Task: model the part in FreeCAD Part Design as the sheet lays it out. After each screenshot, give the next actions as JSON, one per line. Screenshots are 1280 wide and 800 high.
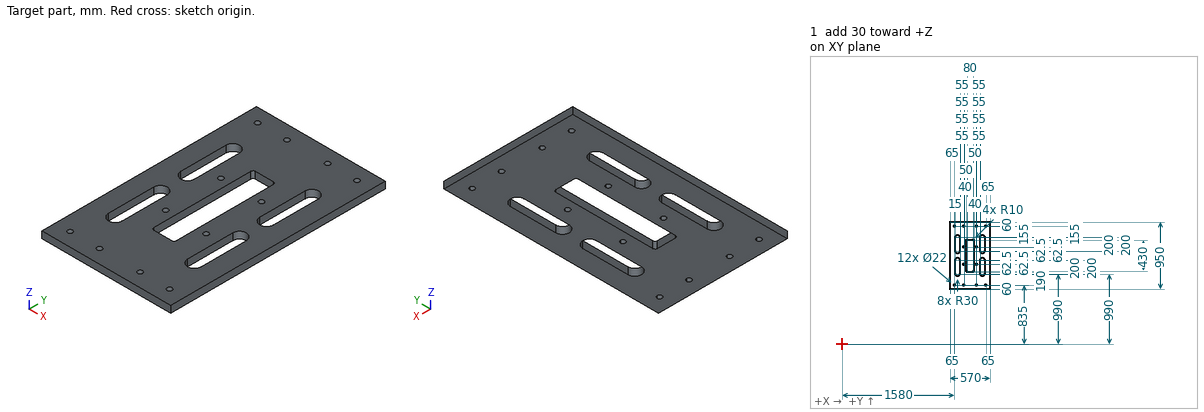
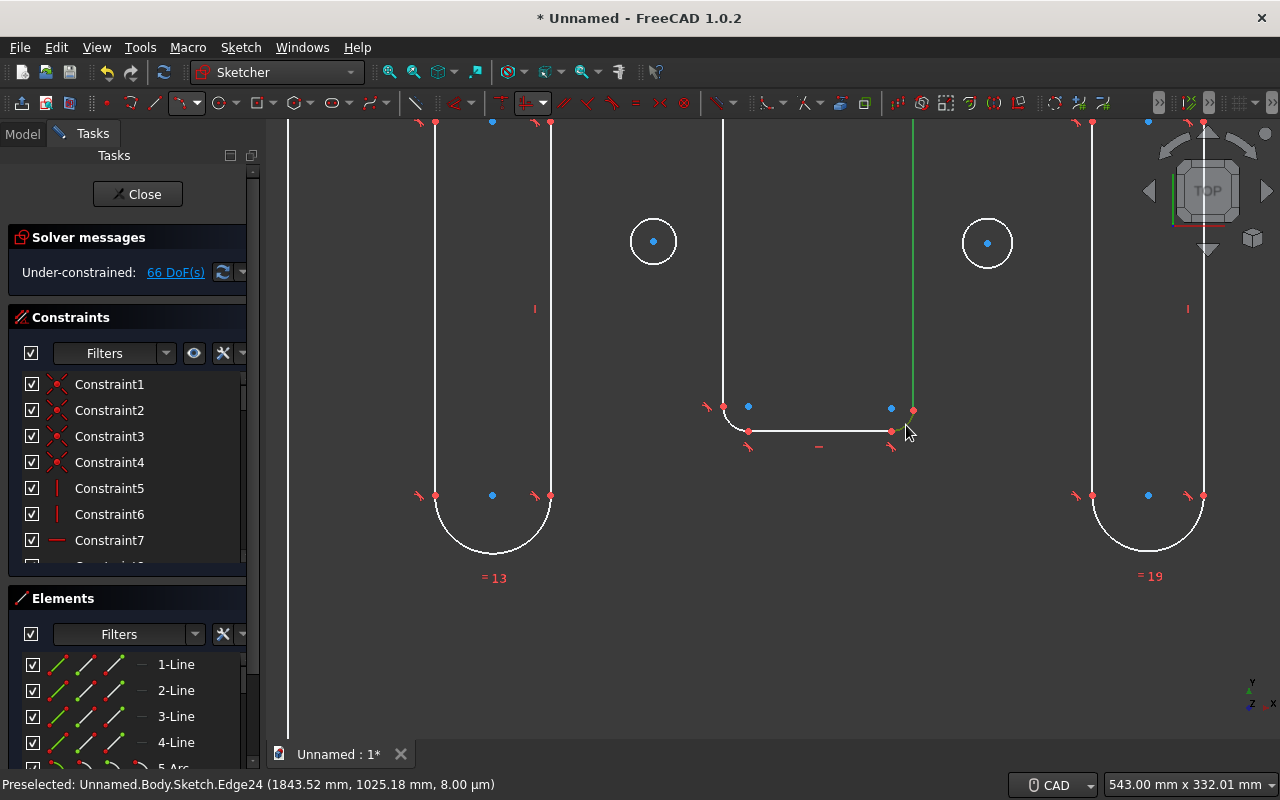
{"action": "left_click", "coordinate": [612, 104]}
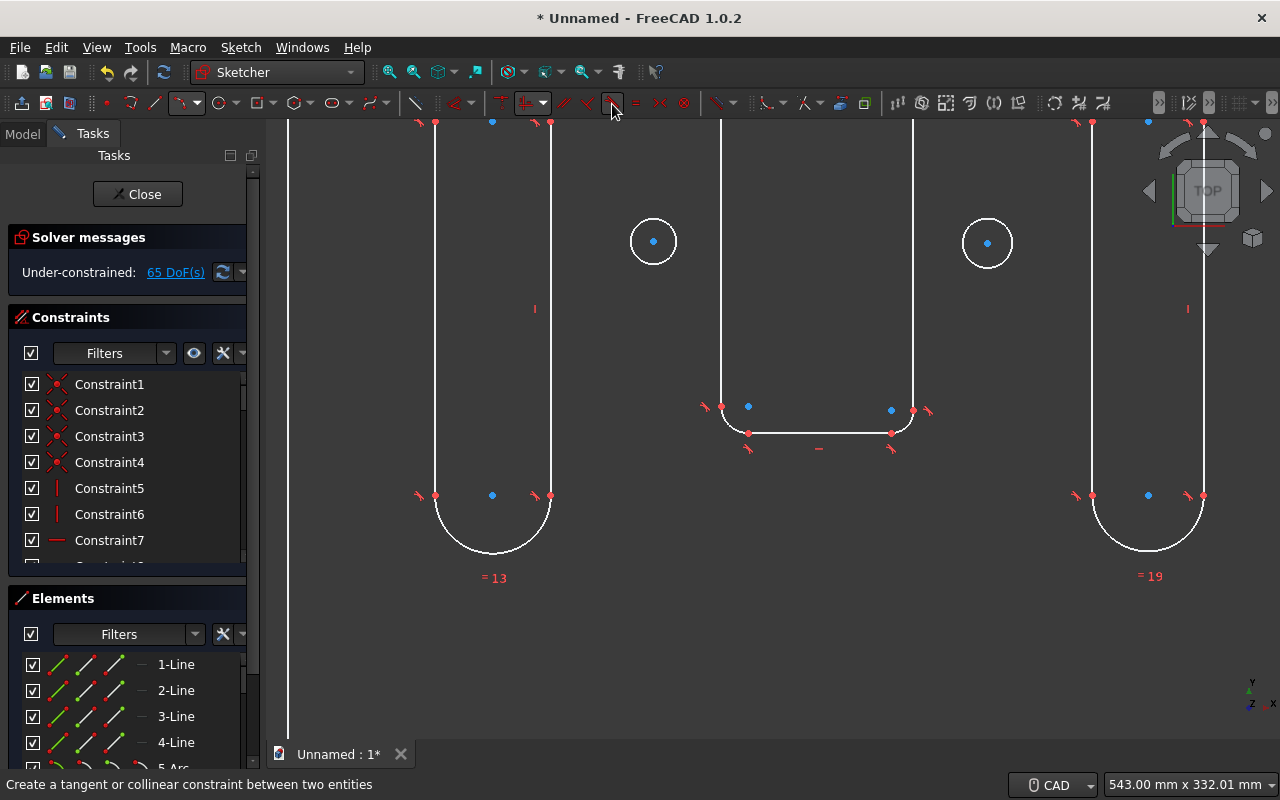
{"action": "scroll", "coordinate": [908, 382], "scroll_direction": "down", "scroll_amount": 10}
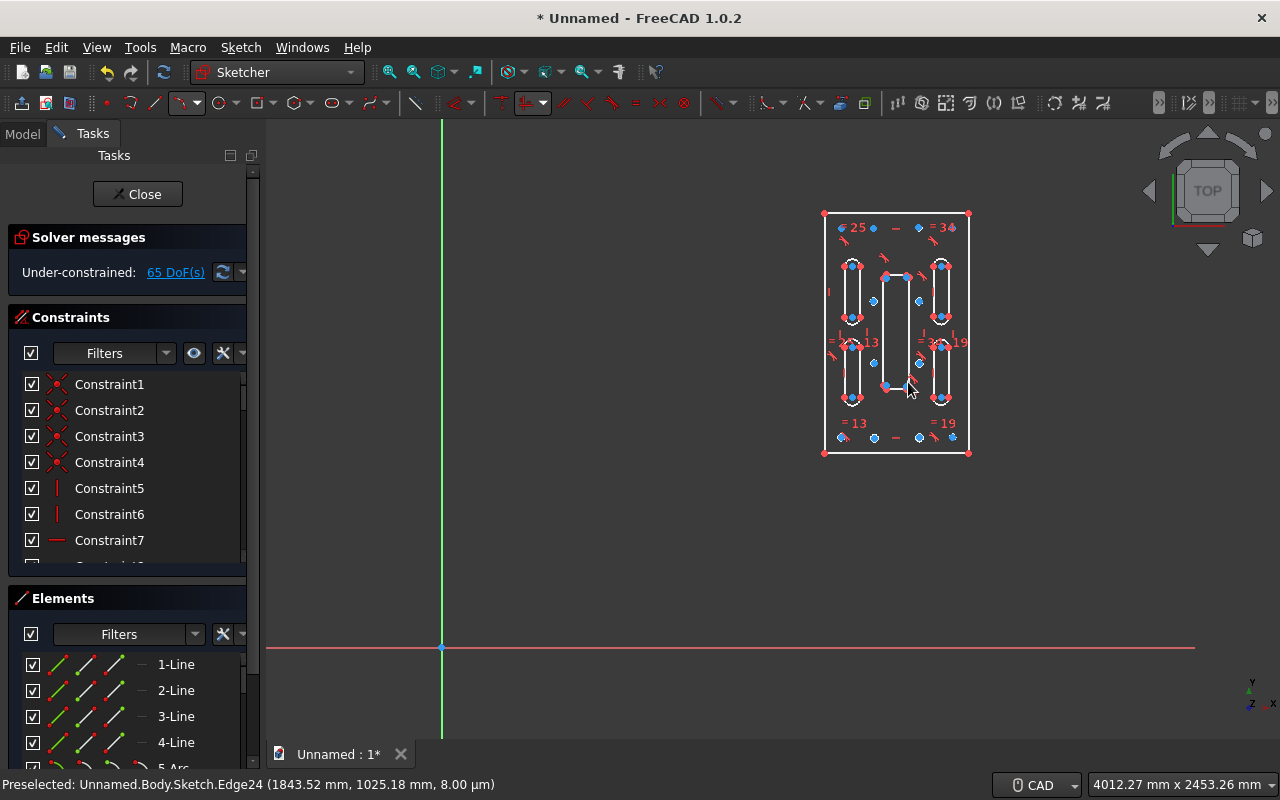
{"action": "scroll", "coordinate": [893, 275], "scroll_direction": "up", "scroll_amount": 5}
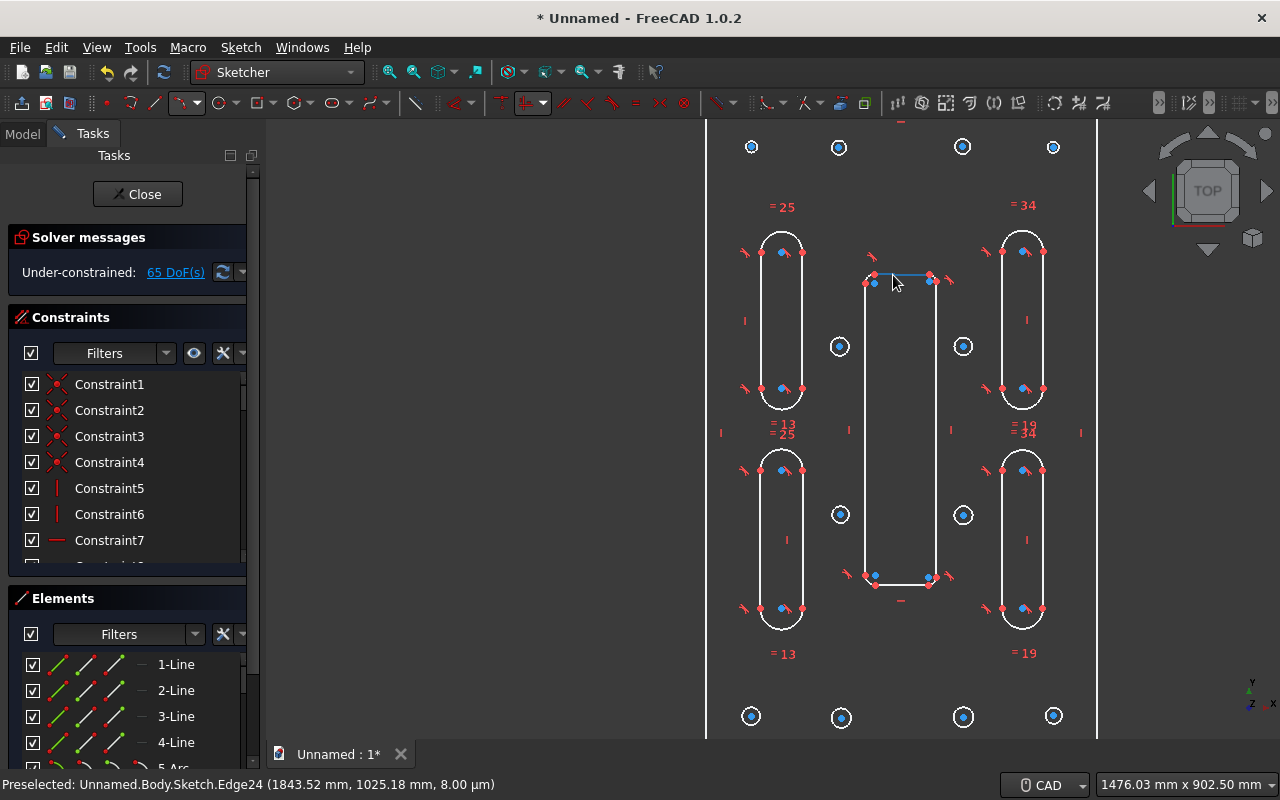
{"action": "left_click", "coordinate": [891, 274]}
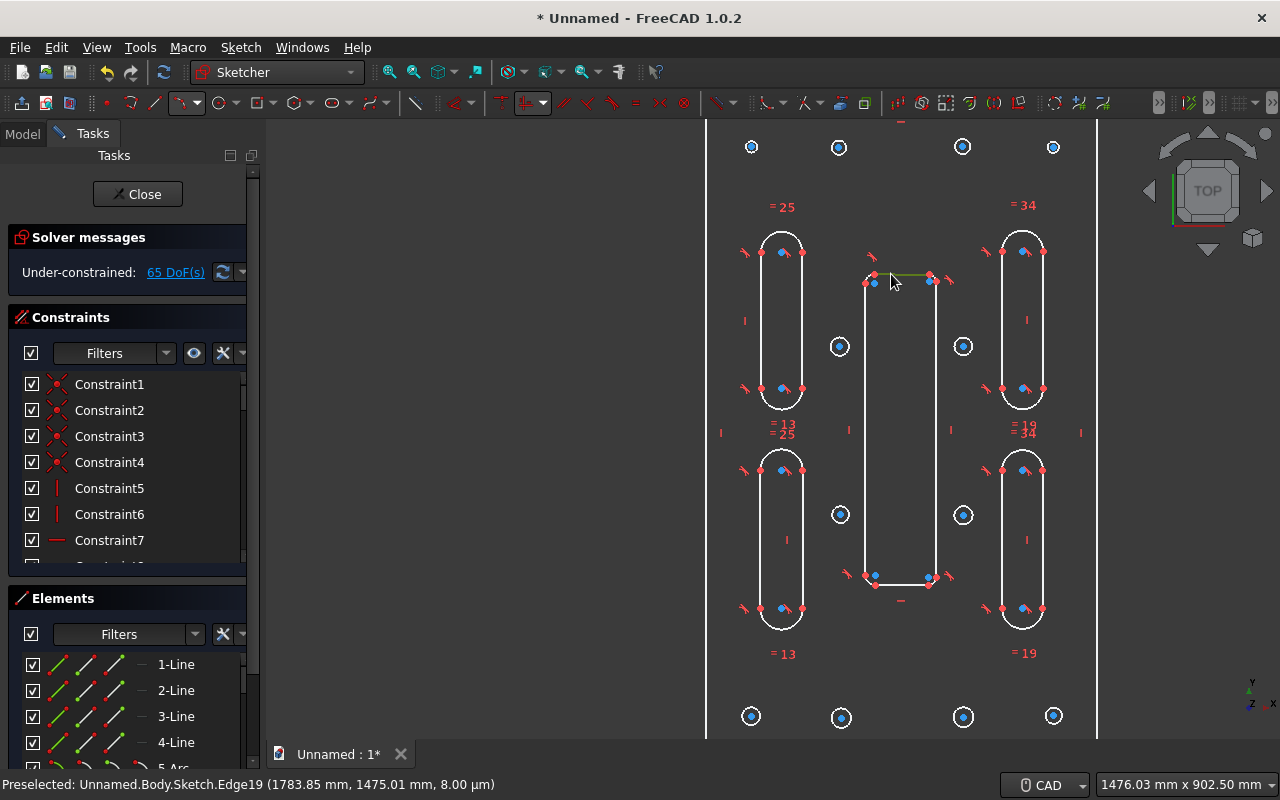
{"action": "left_click", "coordinate": [546, 104]}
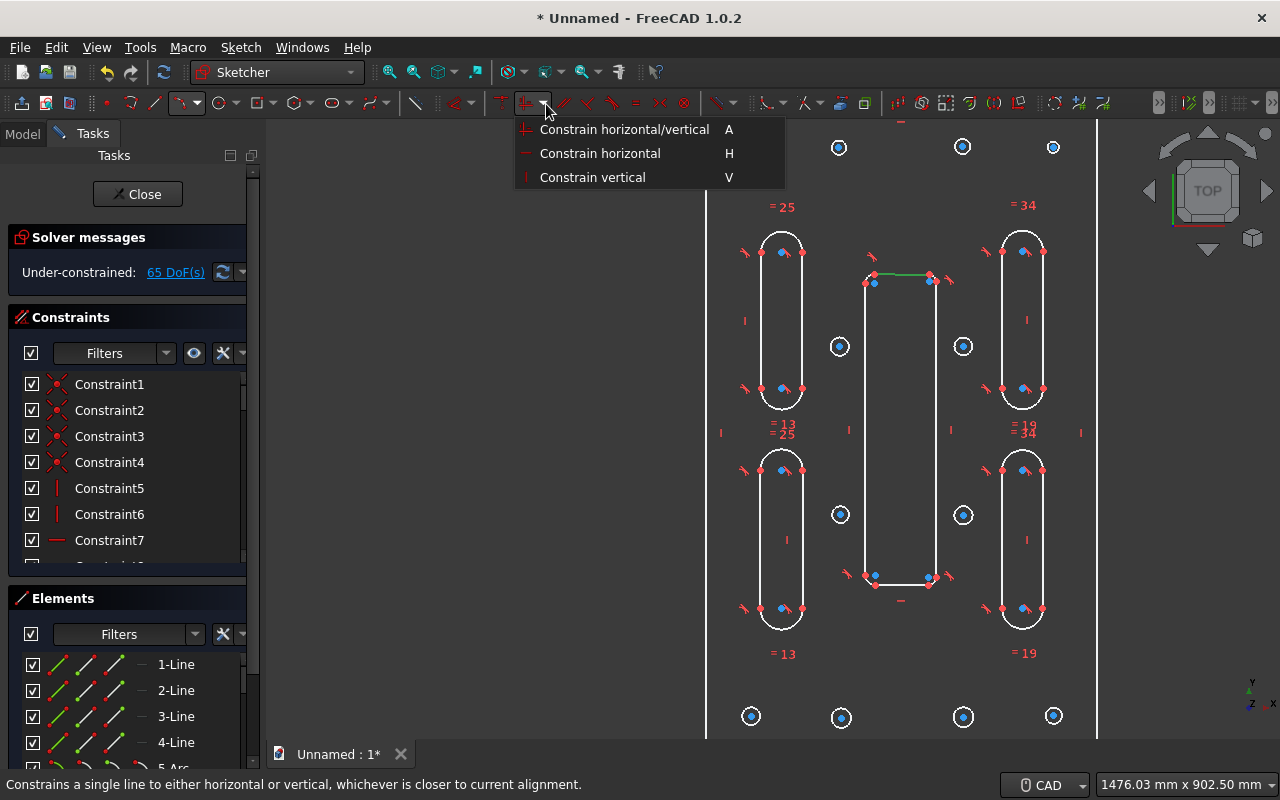
{"action": "left_click", "coordinate": [650, 153]}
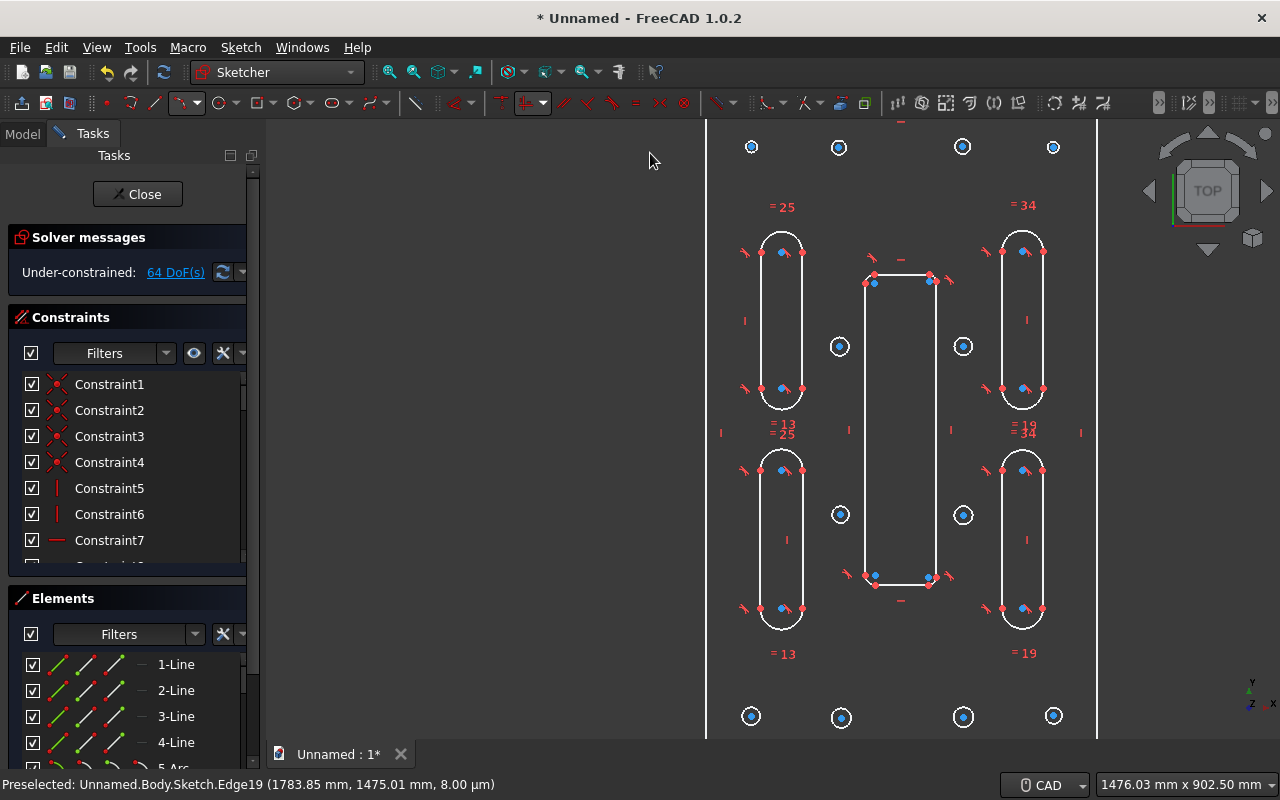
{"action": "left_click", "coordinate": [769, 625]}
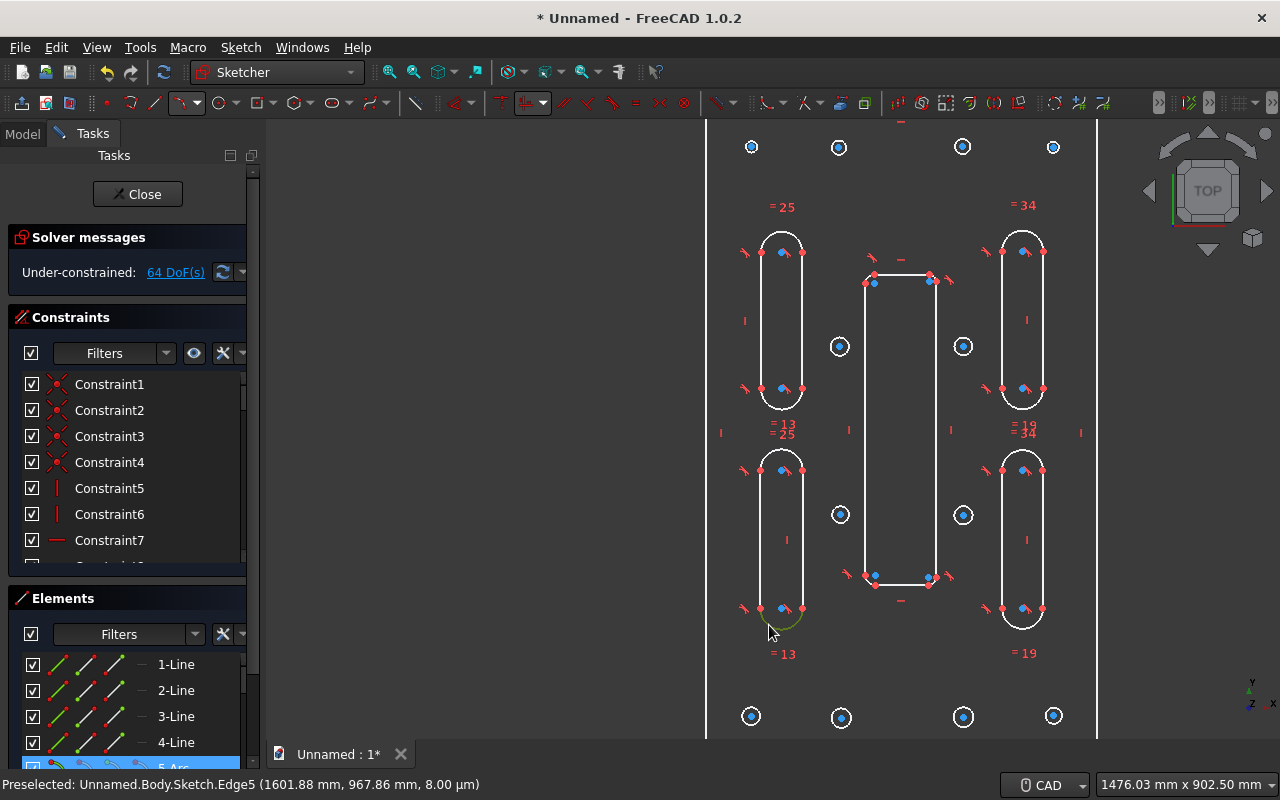
{"action": "left_click", "coordinate": [1010, 625]}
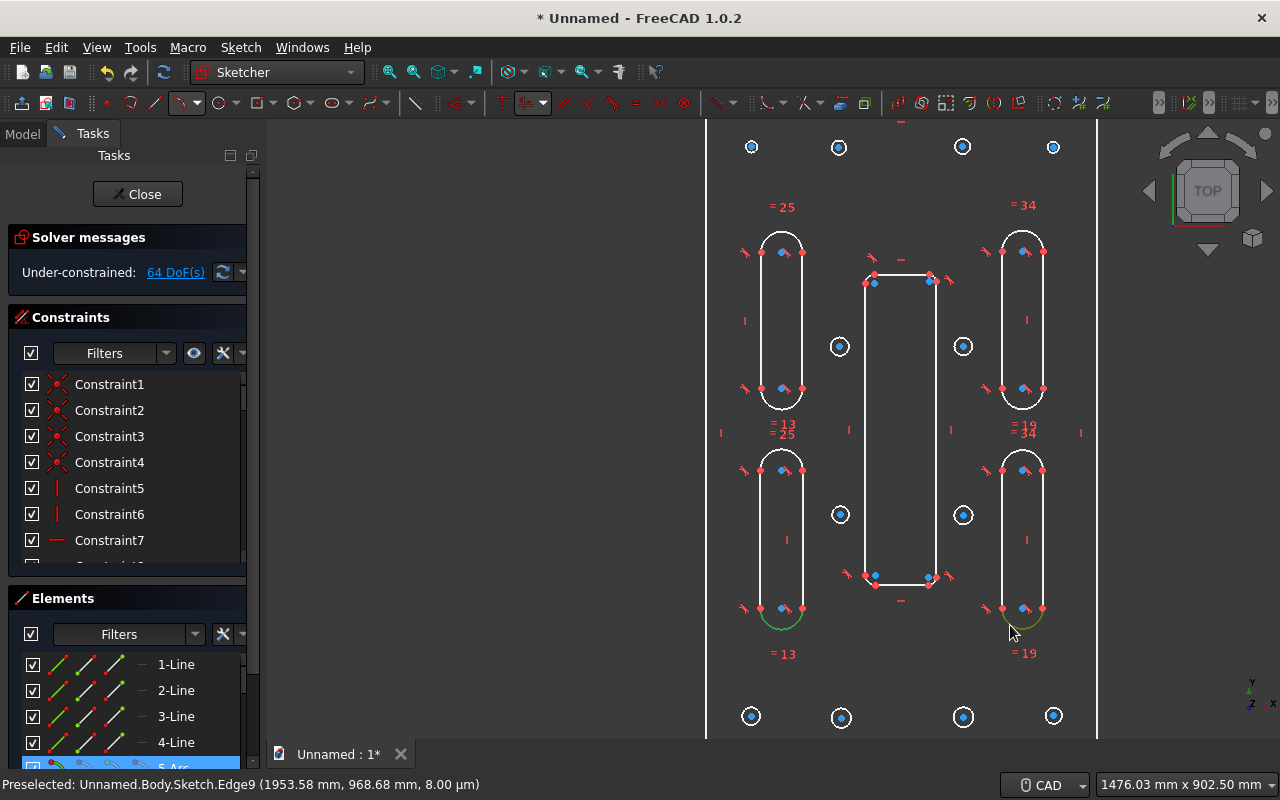
{"action": "left_click", "coordinate": [770, 406]}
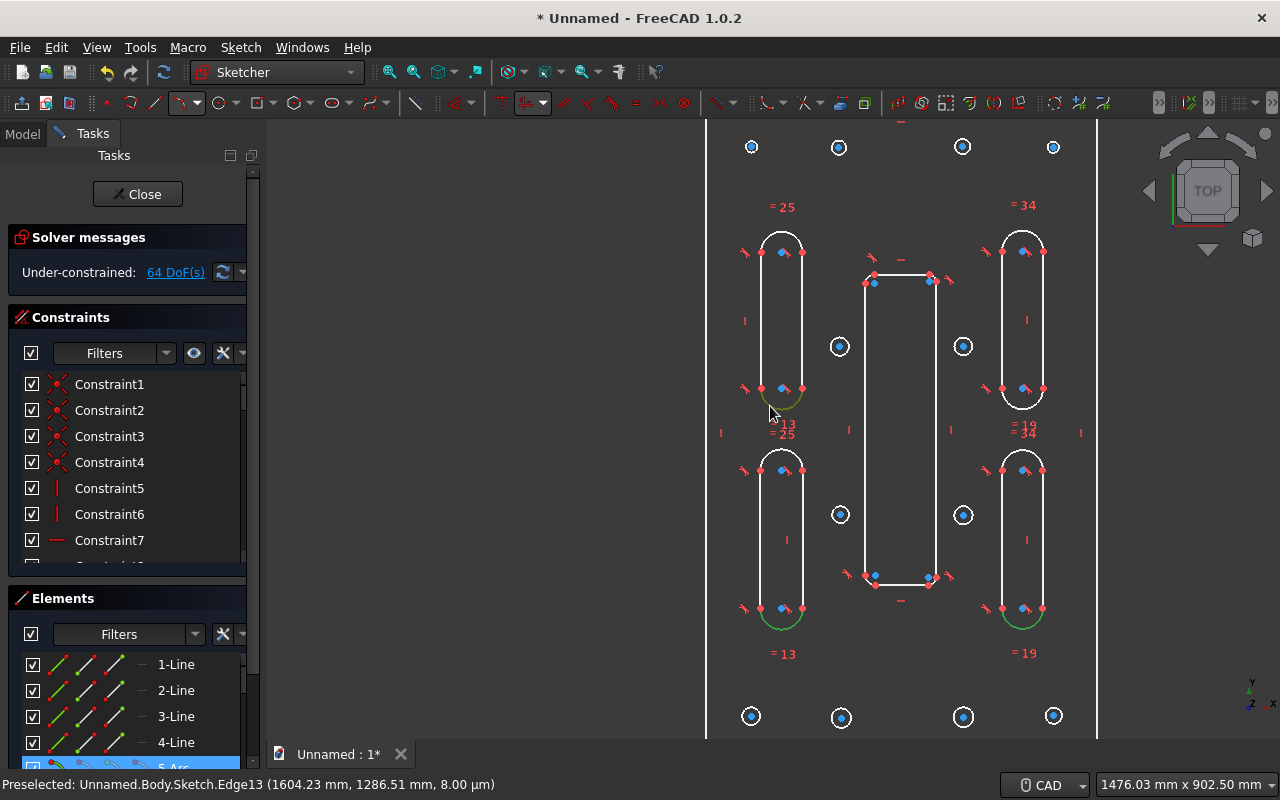
{"action": "left_click", "coordinate": [1011, 405]}